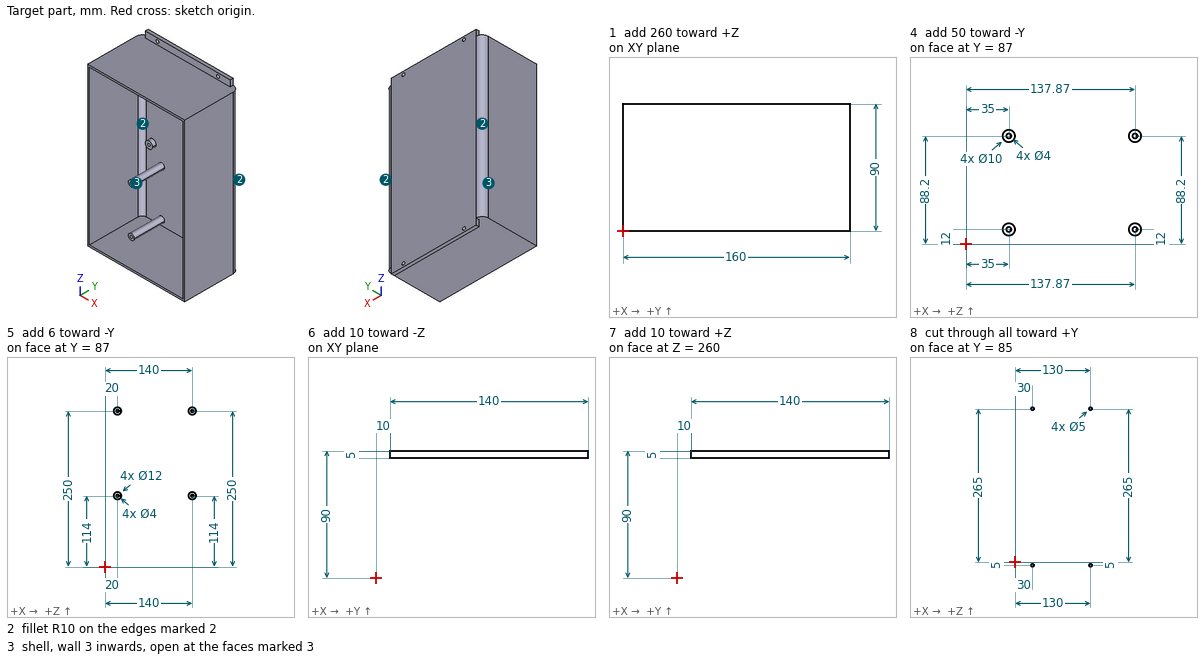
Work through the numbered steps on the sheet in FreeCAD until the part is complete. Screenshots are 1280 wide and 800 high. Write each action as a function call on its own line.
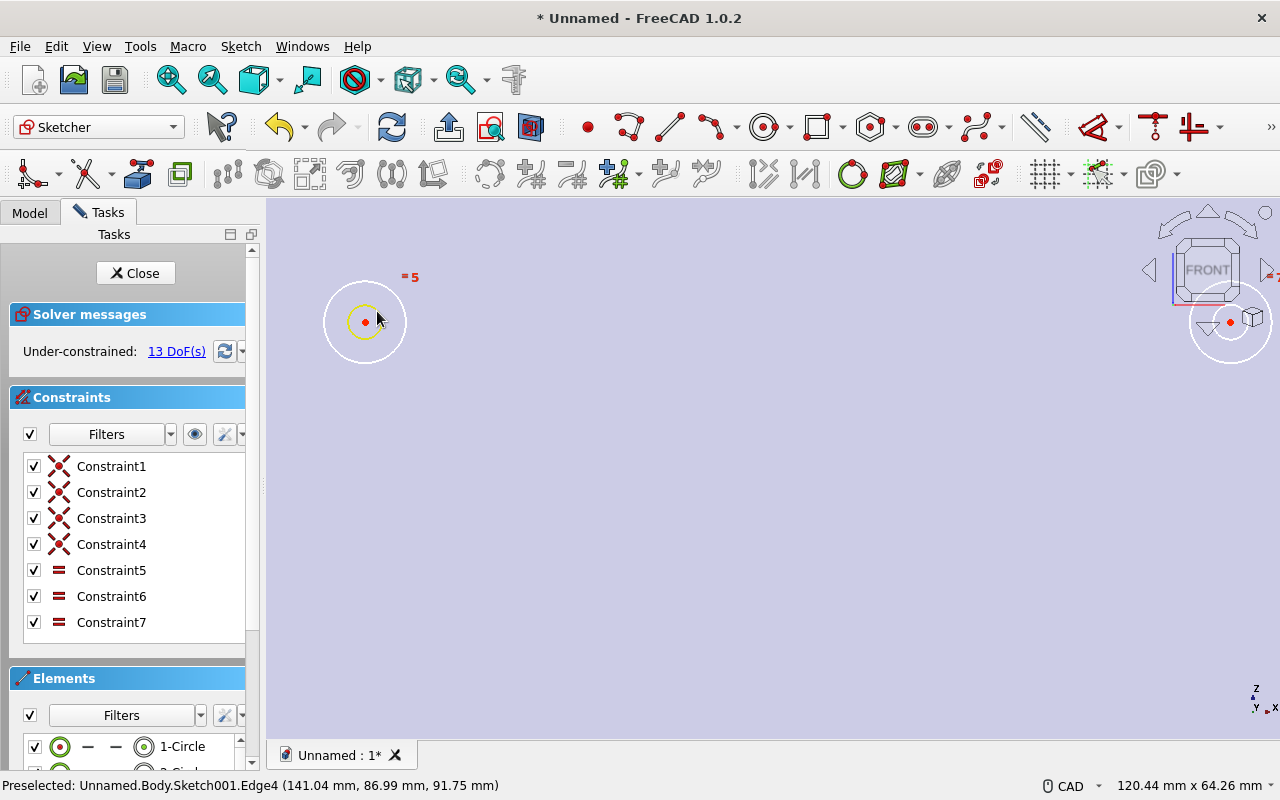
click(377, 310)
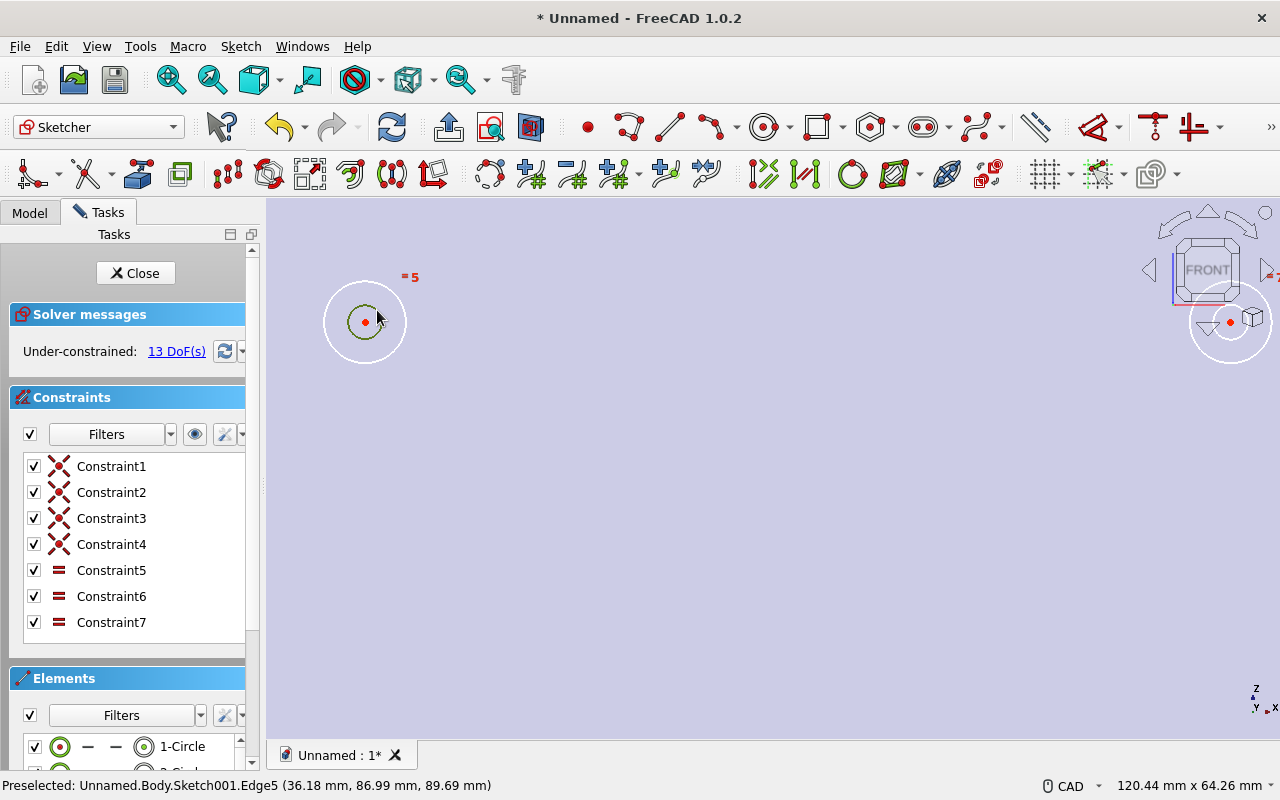
scroll(732, 303, down, 4)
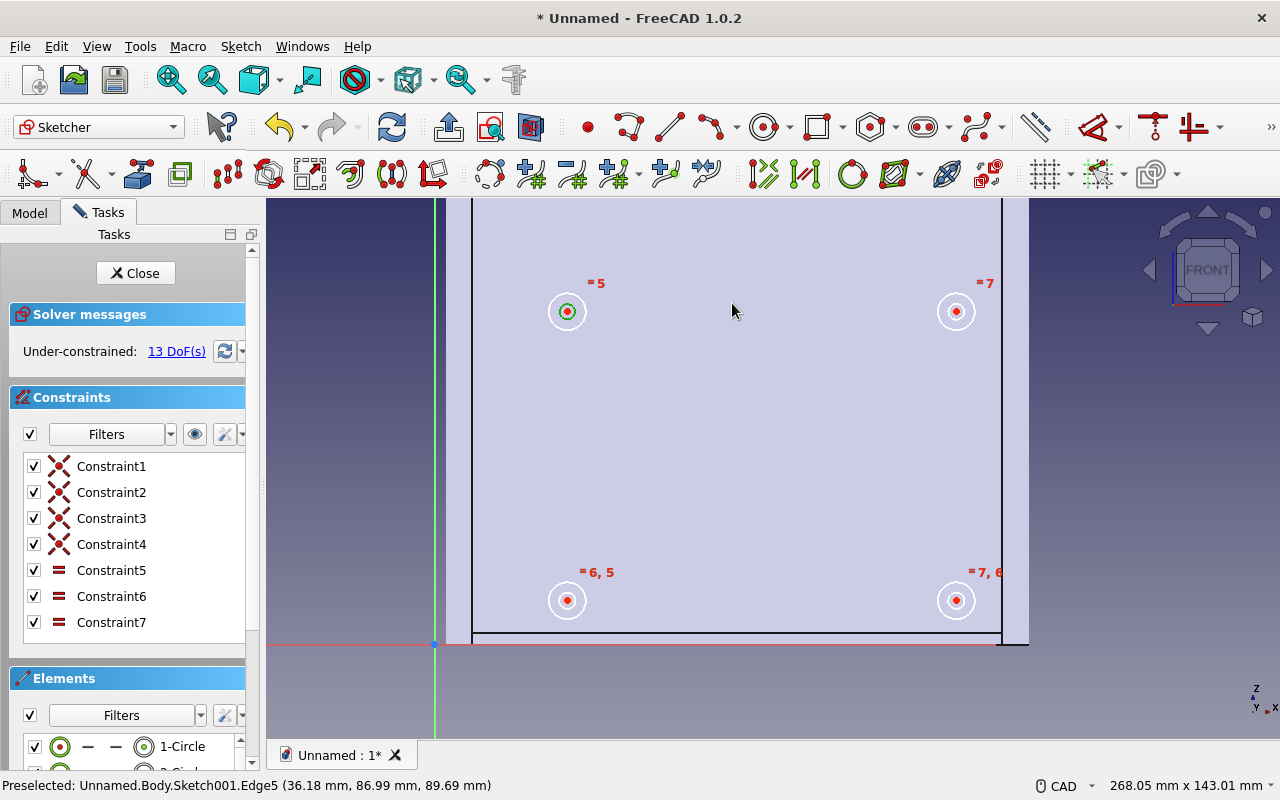
scroll(573, 595, up, 3)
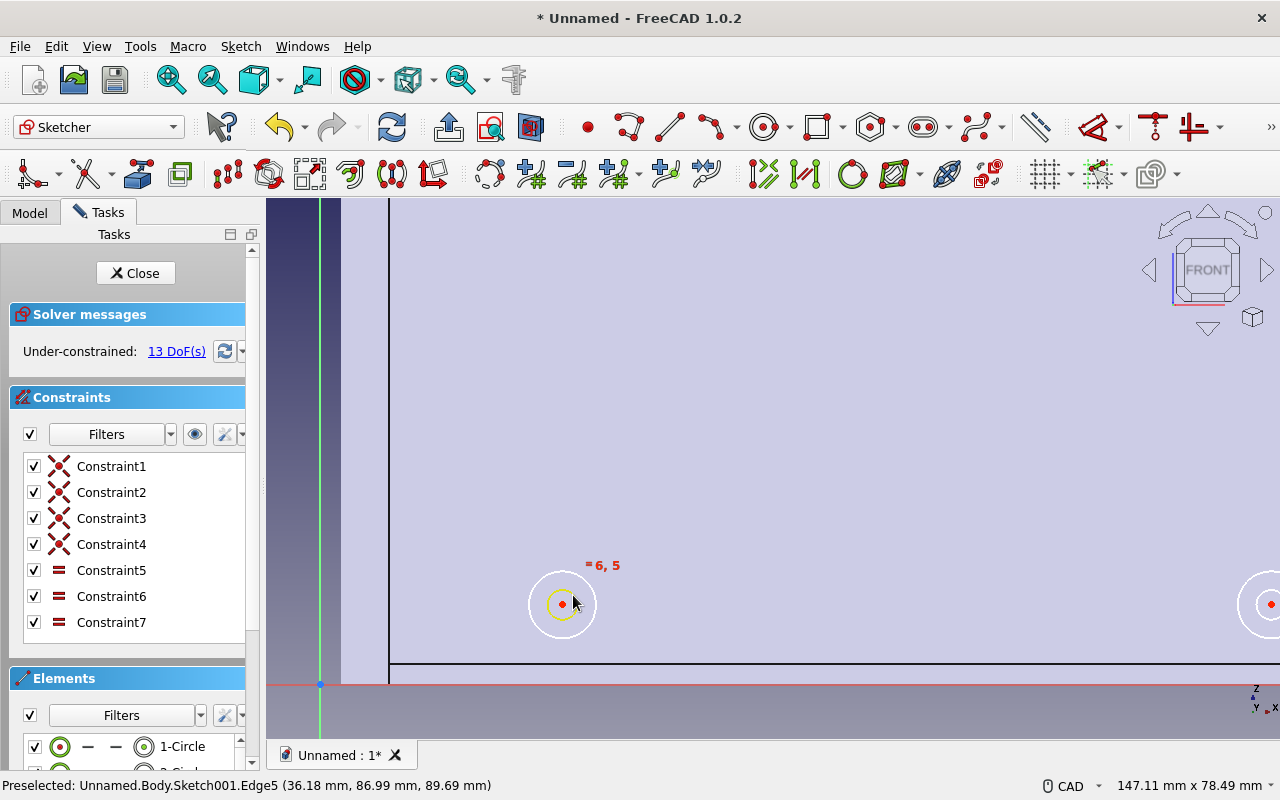
click(573, 594)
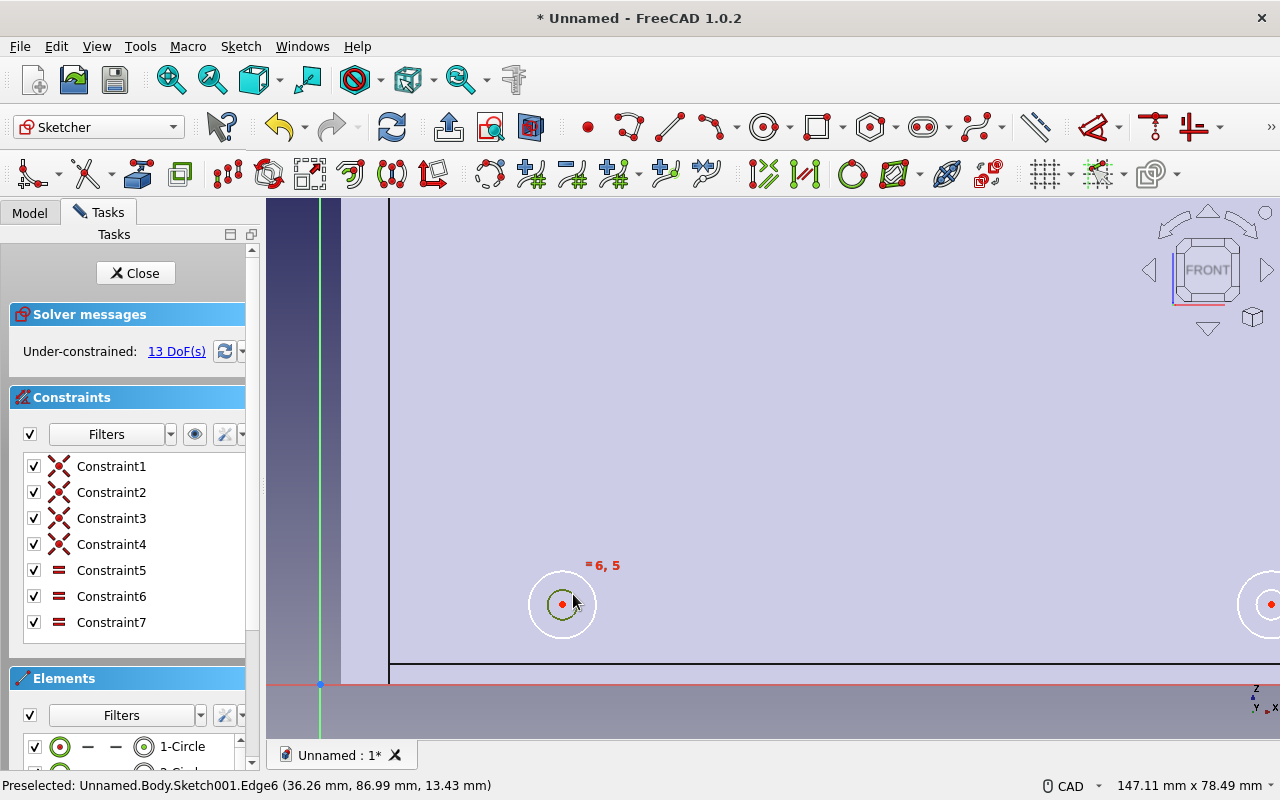
scroll(573, 596, down, 3)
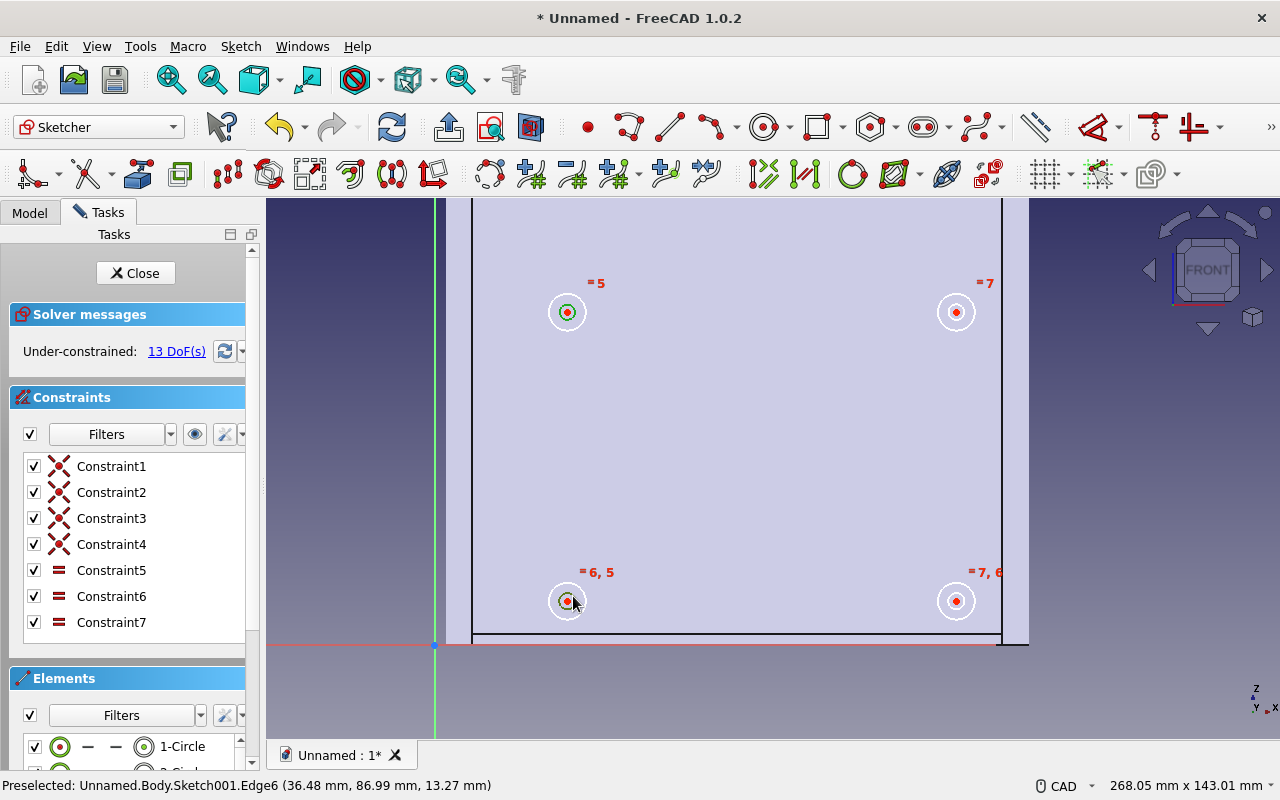
scroll(962, 595, up, 3)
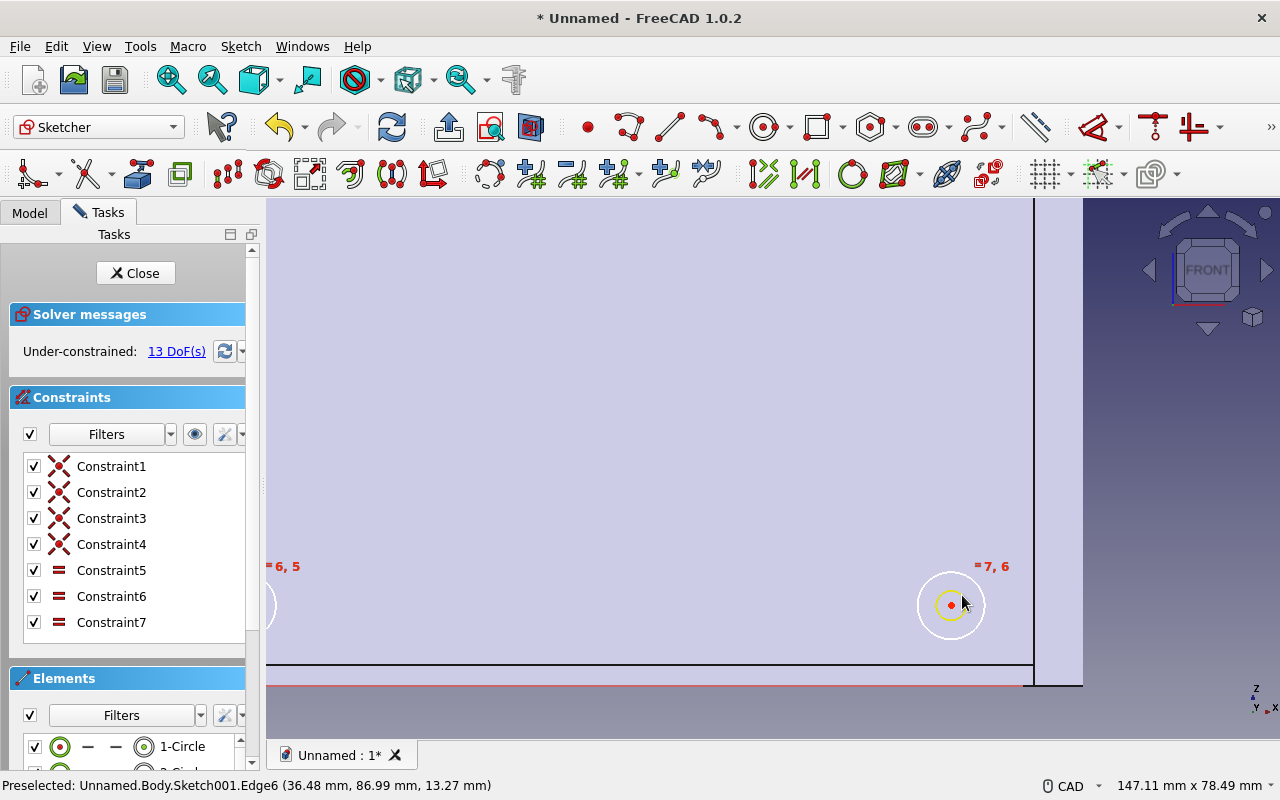
click(962, 595)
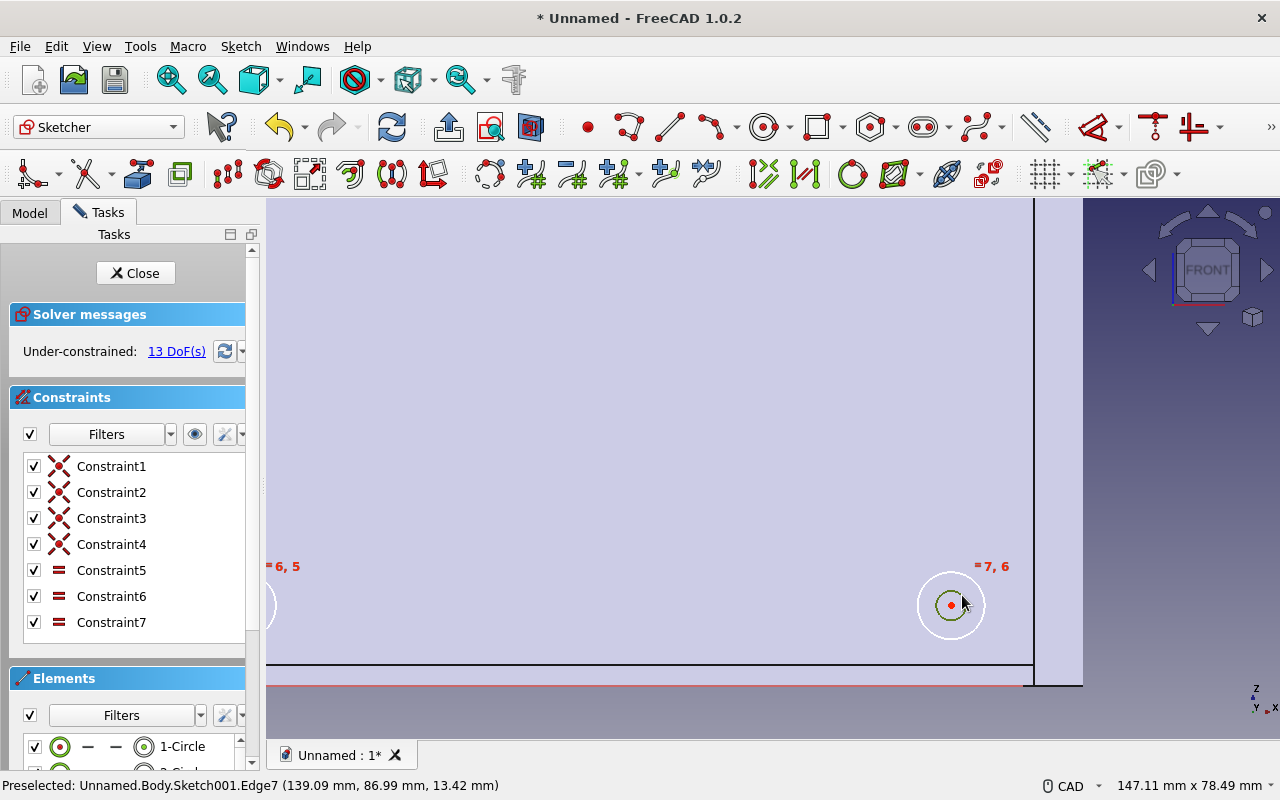
scroll(962, 595, down, 3)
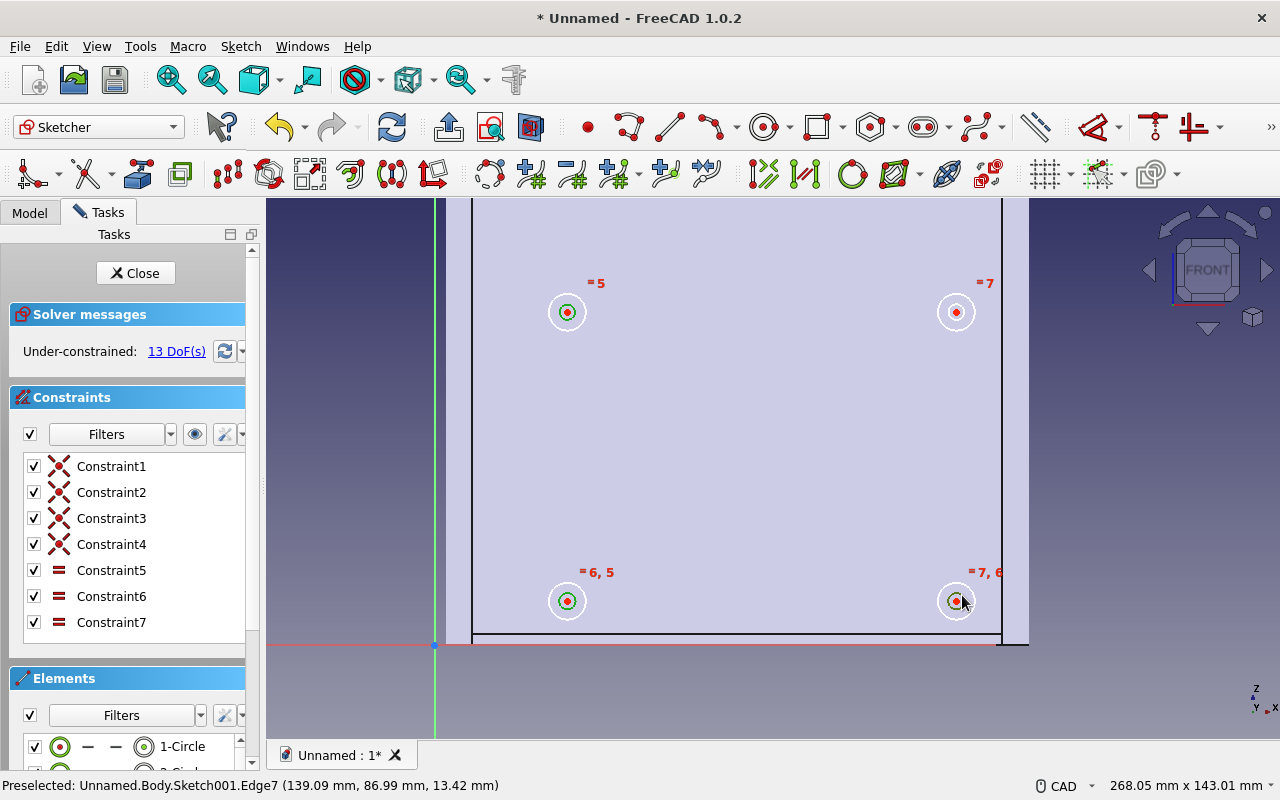
scroll(962, 307, up, 3)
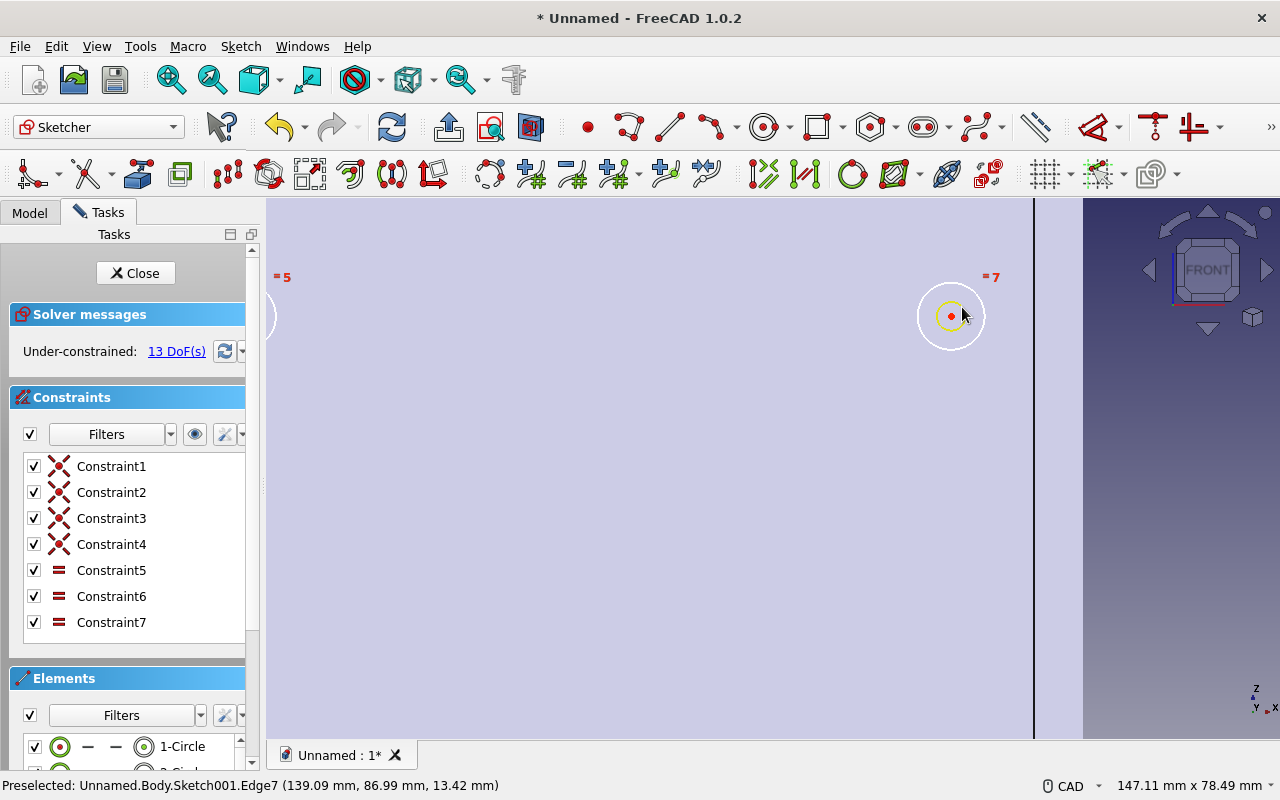
click(961, 306)